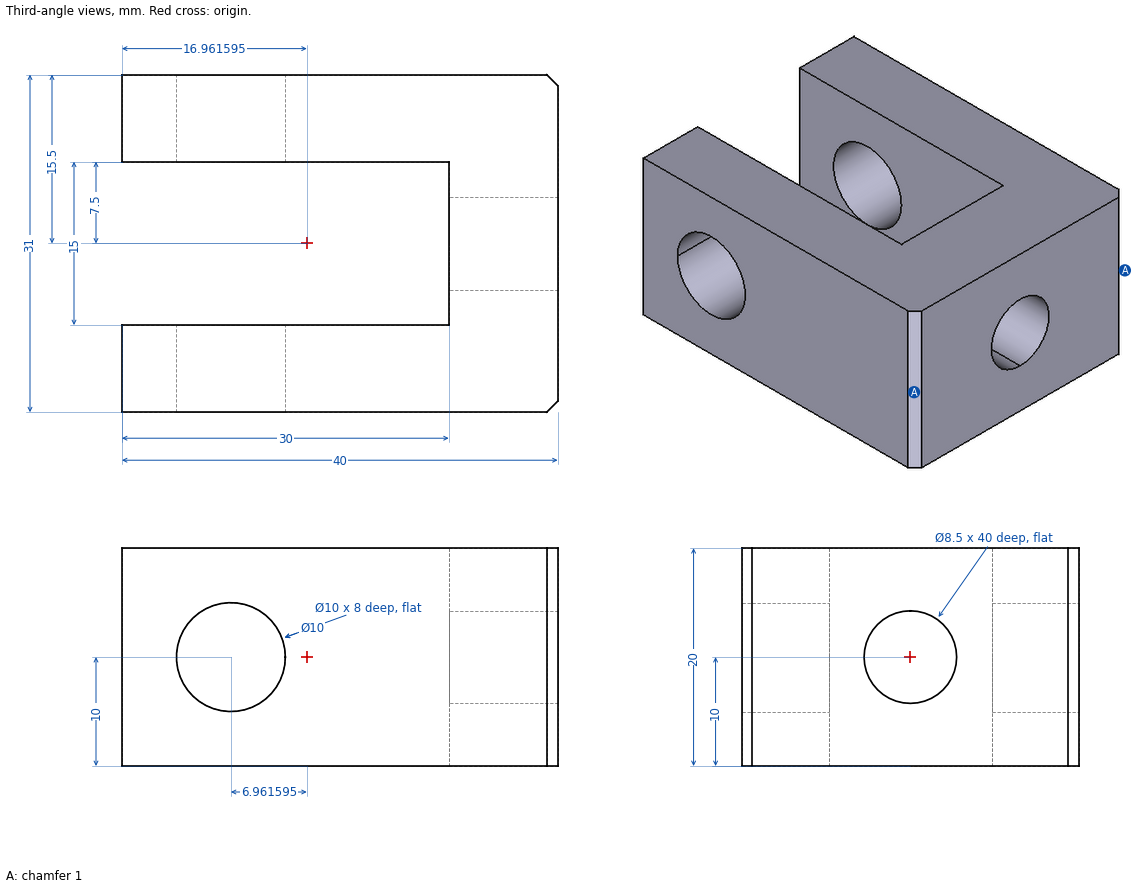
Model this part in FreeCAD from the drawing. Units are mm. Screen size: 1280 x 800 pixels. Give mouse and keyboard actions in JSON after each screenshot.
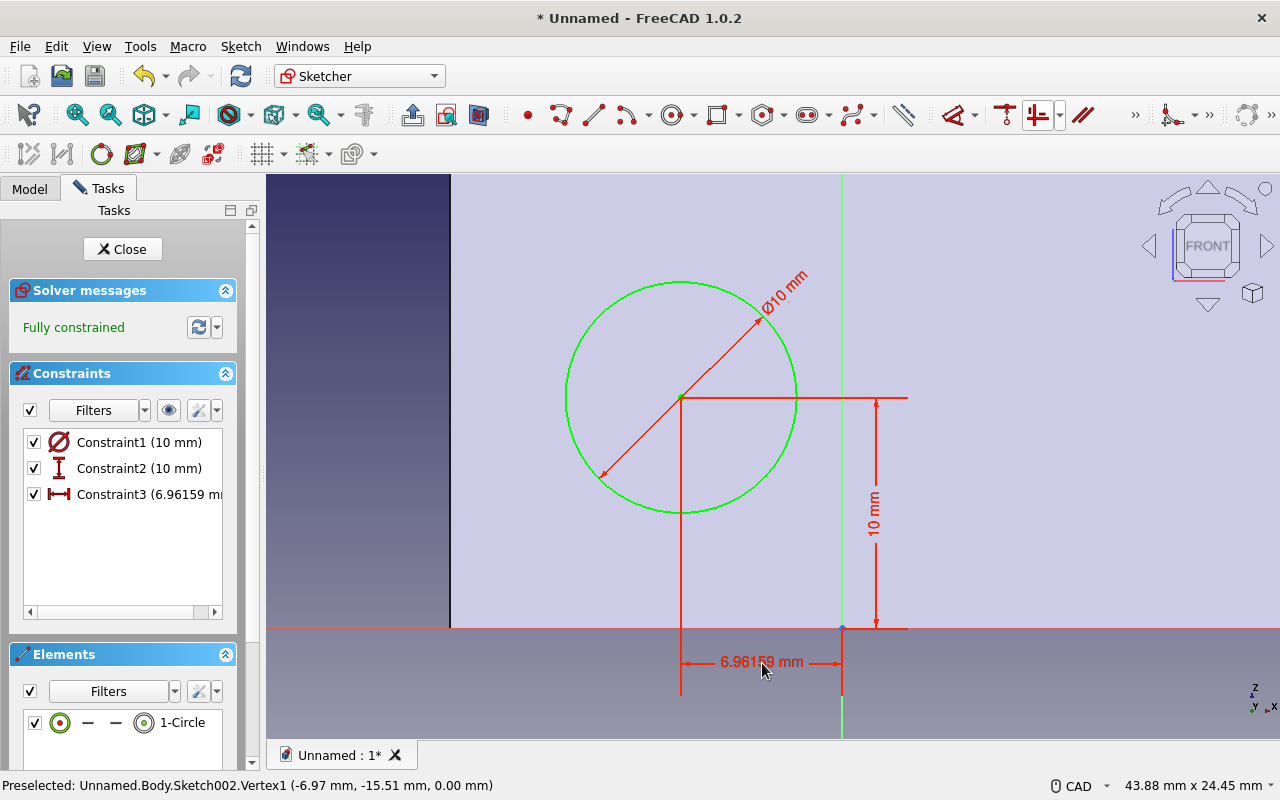
{"action": "left_click", "coordinate": [123, 249]}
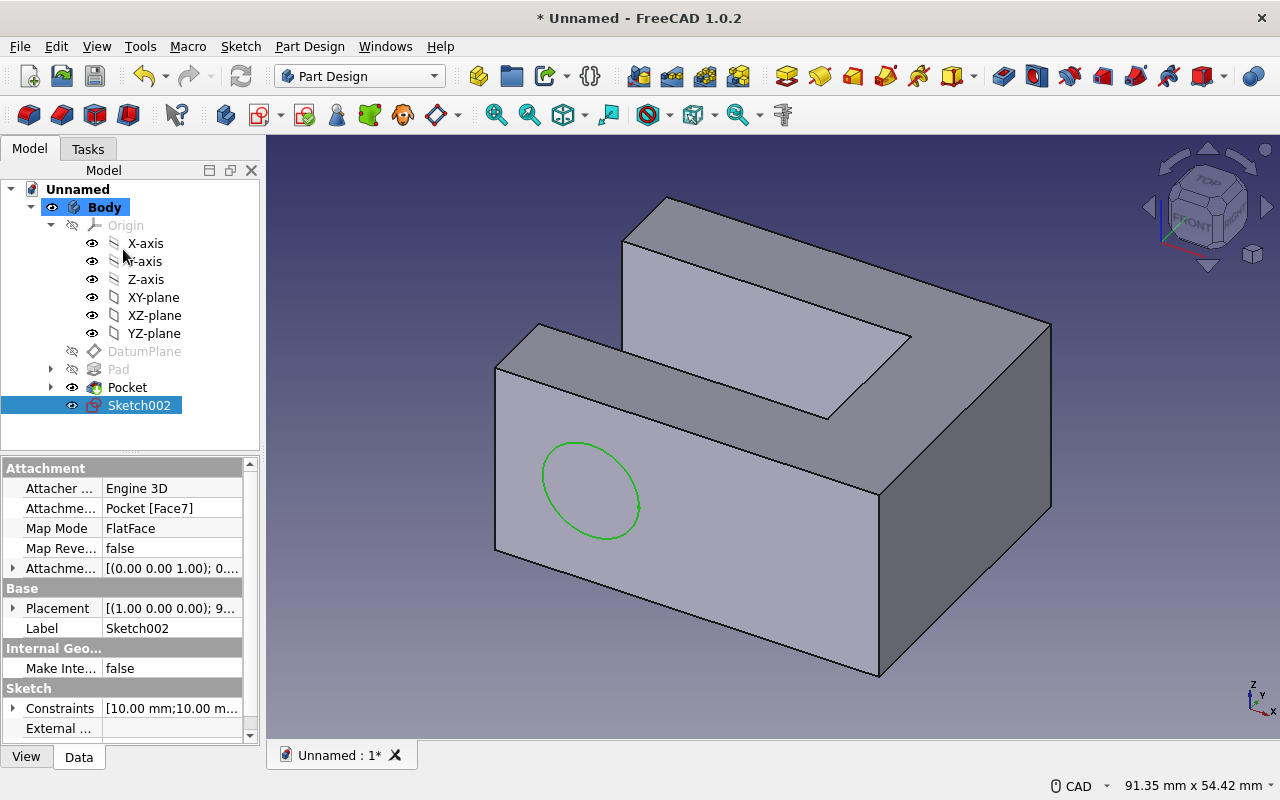
{"action": "left_click", "coordinate": [1037, 76]}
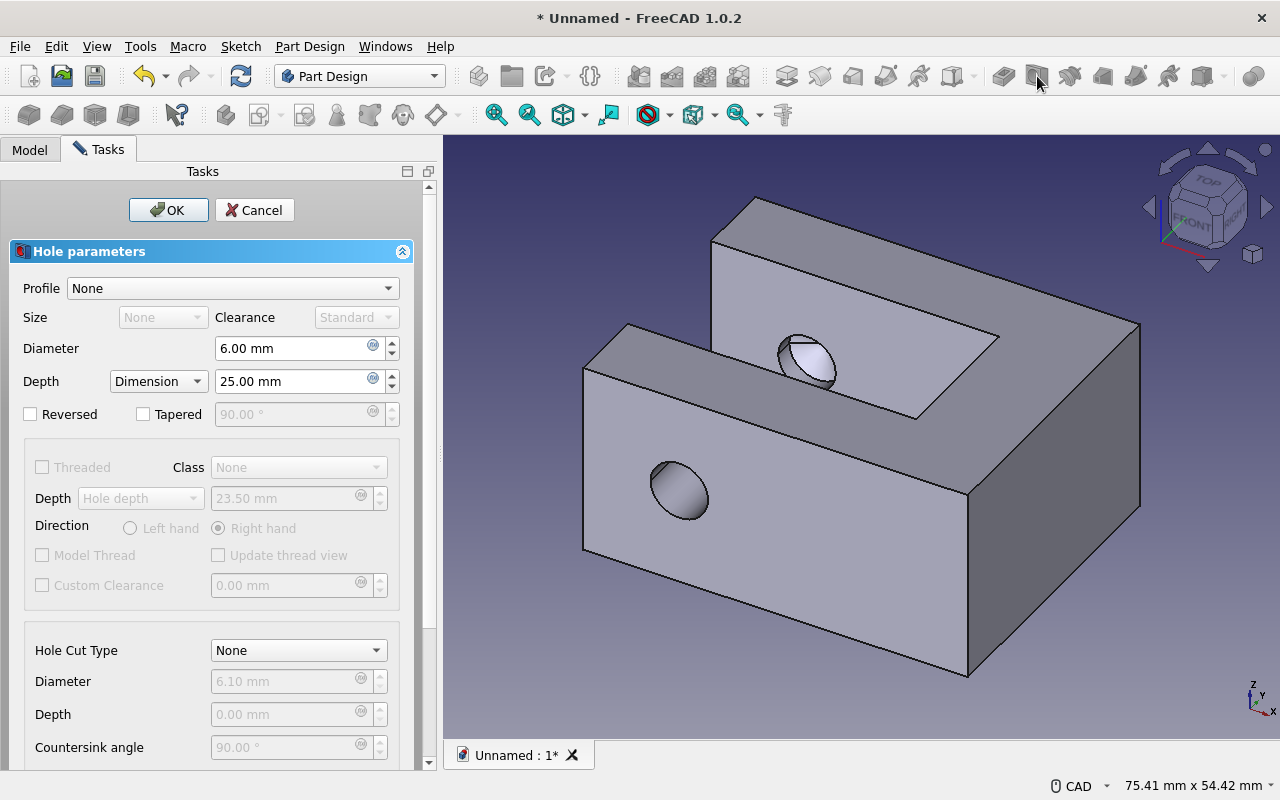
{"action": "triple_click", "coordinate": [300, 348]}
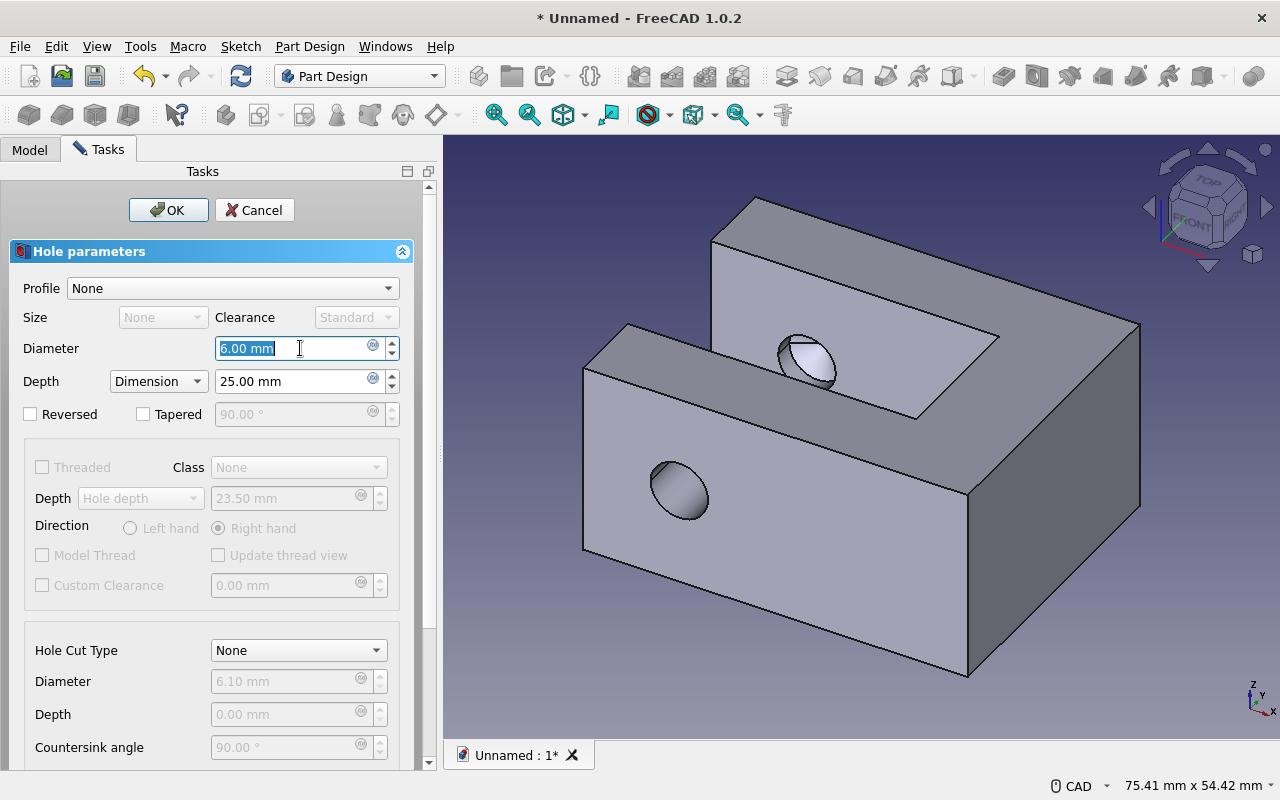
{"action": "type", "text": "10"}
{"action": "key", "text": "Tab"}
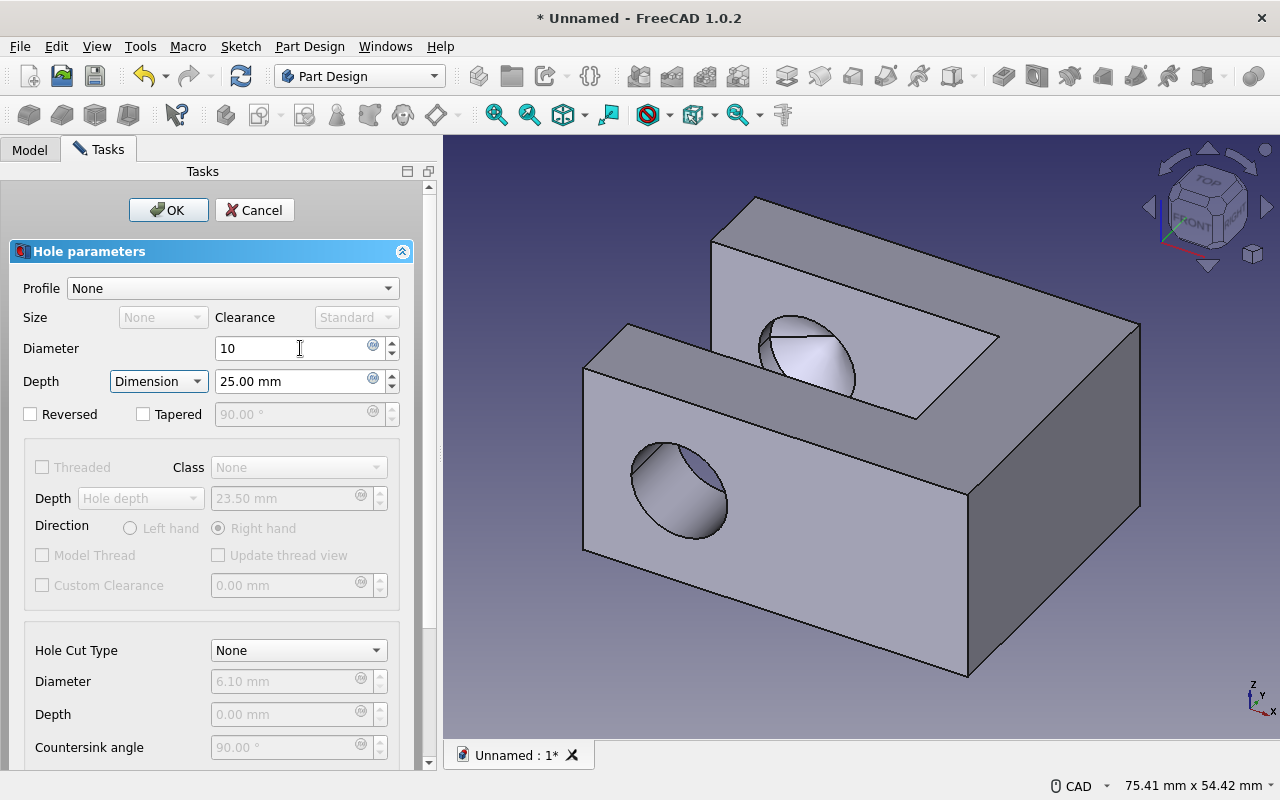
{"action": "triple_click", "coordinate": [300, 382]}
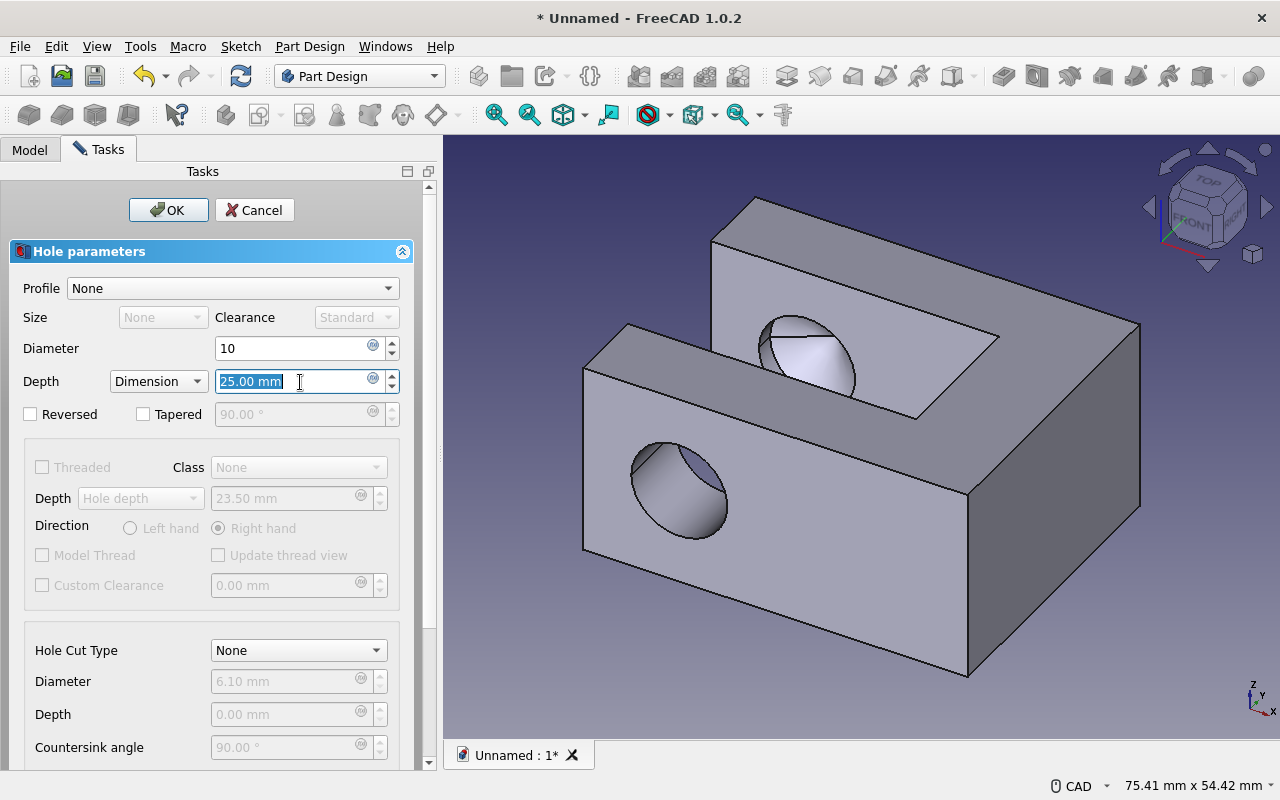
{"action": "type", "text": "8"}
{"action": "key", "text": "Tab"}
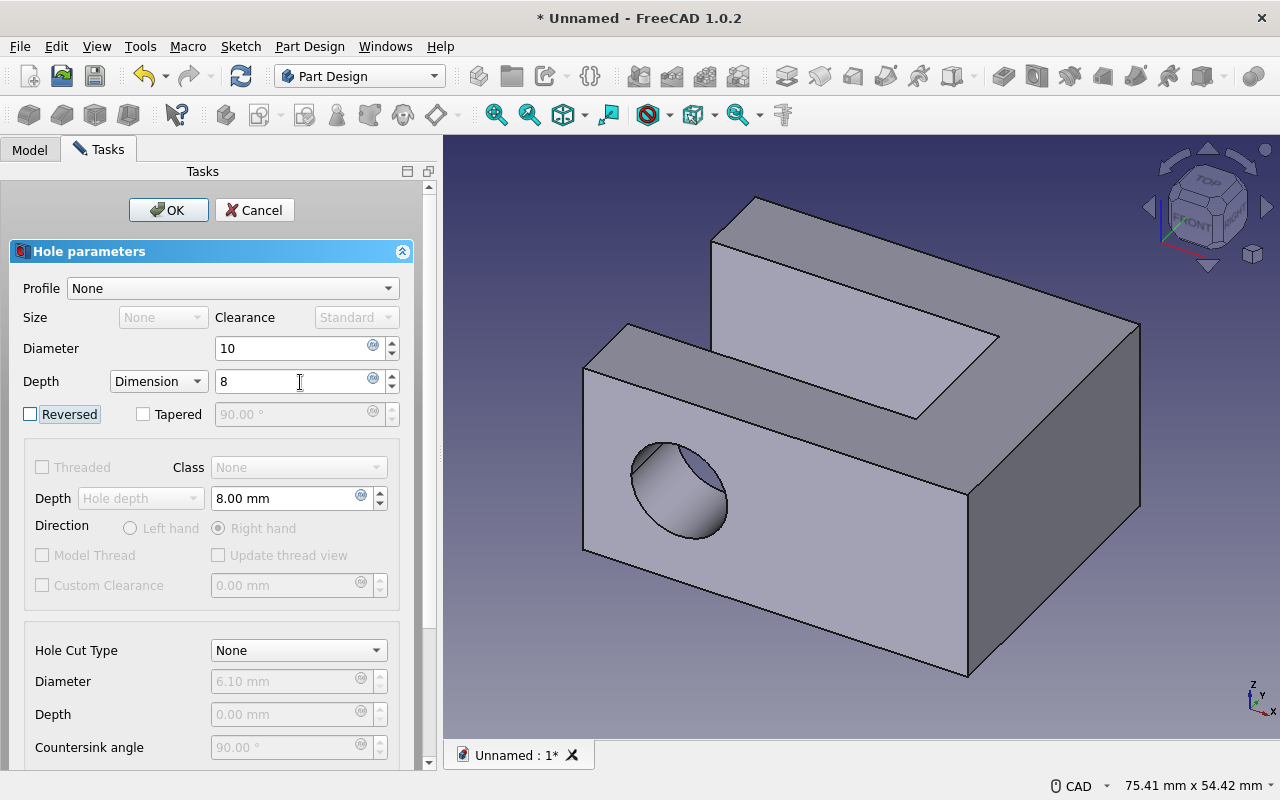
{"action": "scroll", "coordinate": [429, 476], "scroll_direction": "down", "scroll_amount": 3}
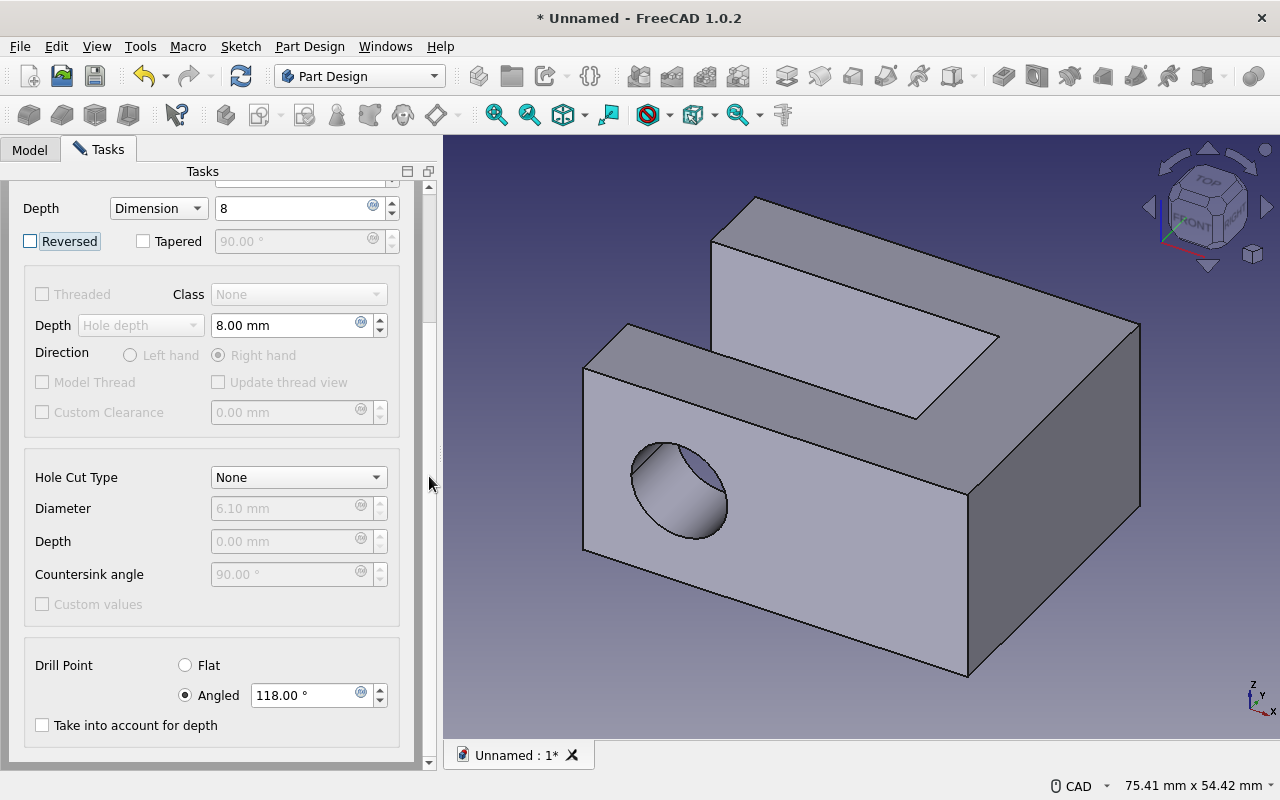
{"action": "left_click", "coordinate": [186, 663]}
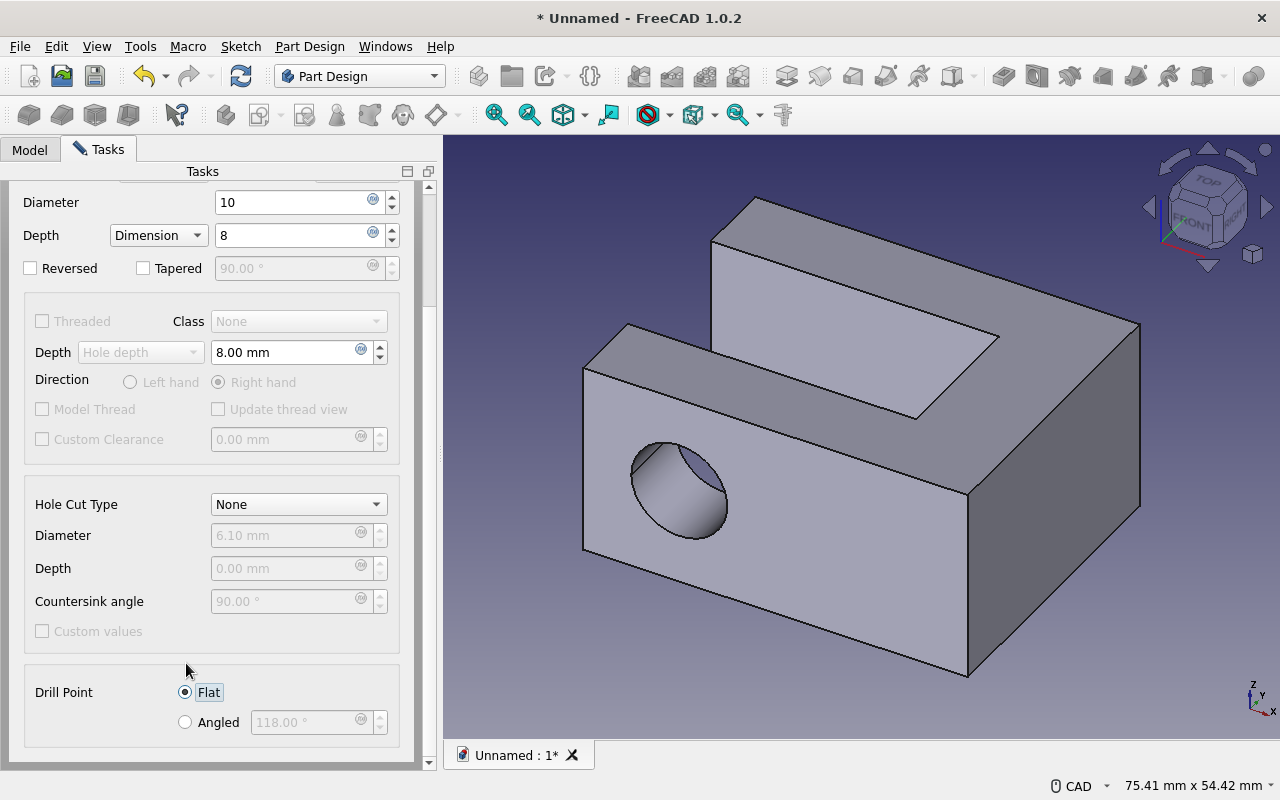
{"action": "scroll", "coordinate": [429, 476], "scroll_direction": "up", "scroll_amount": 4}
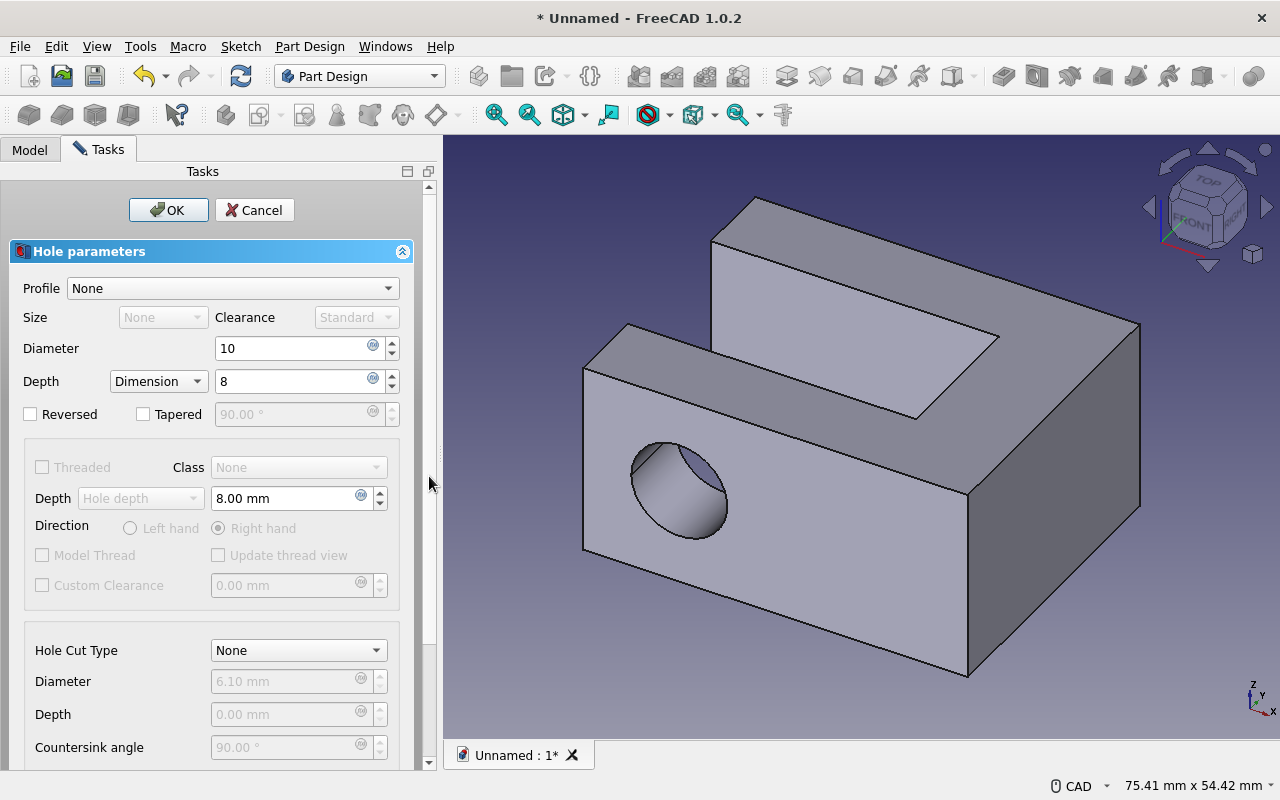
{"action": "left_click", "coordinate": [169, 210]}